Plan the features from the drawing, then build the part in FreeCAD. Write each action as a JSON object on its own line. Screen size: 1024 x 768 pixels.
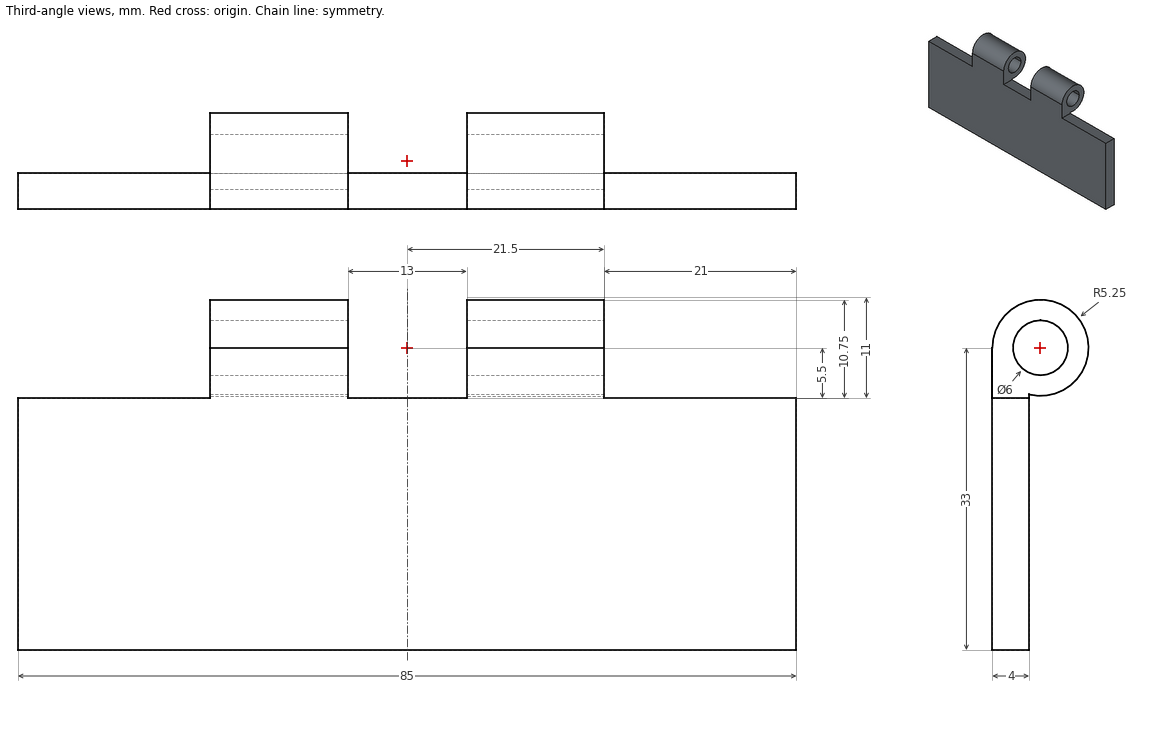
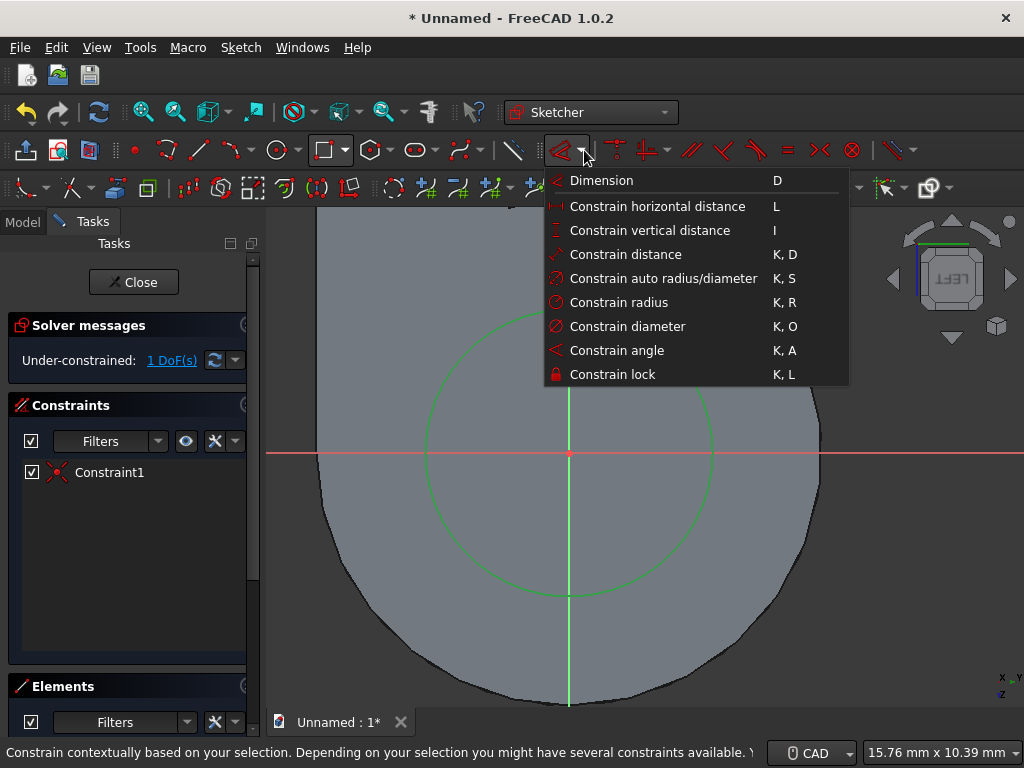
{"action": "left_click", "coordinate": [697, 326]}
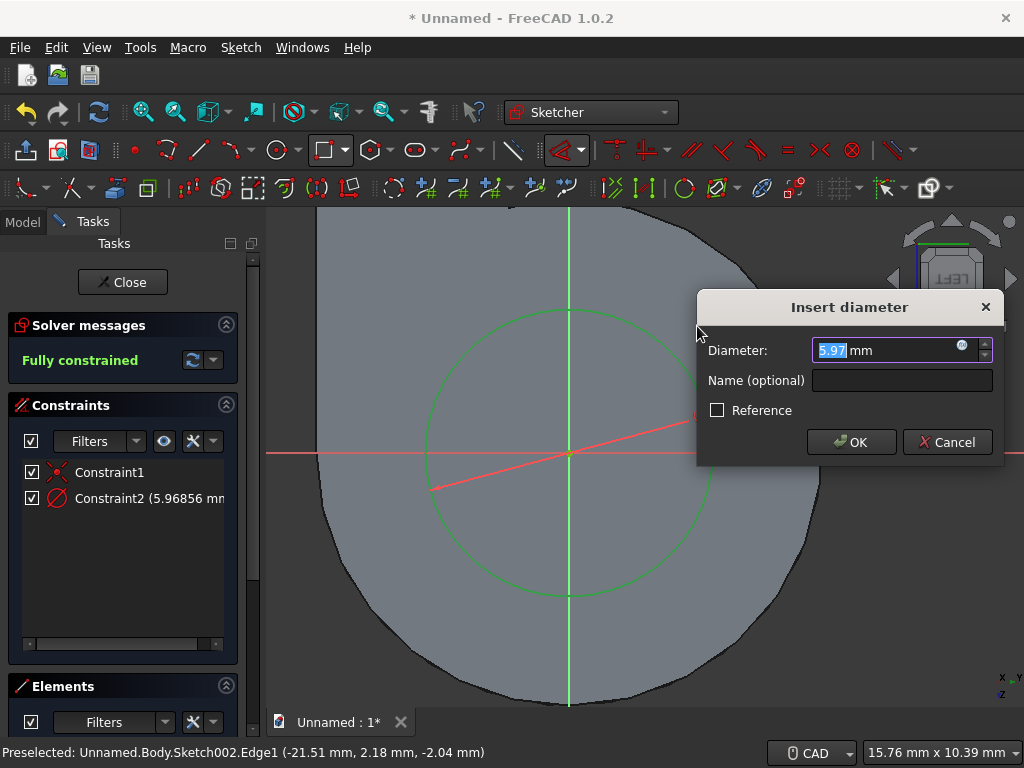
{"action": "type", "text": "6"}
{"action": "key", "text": "Return"}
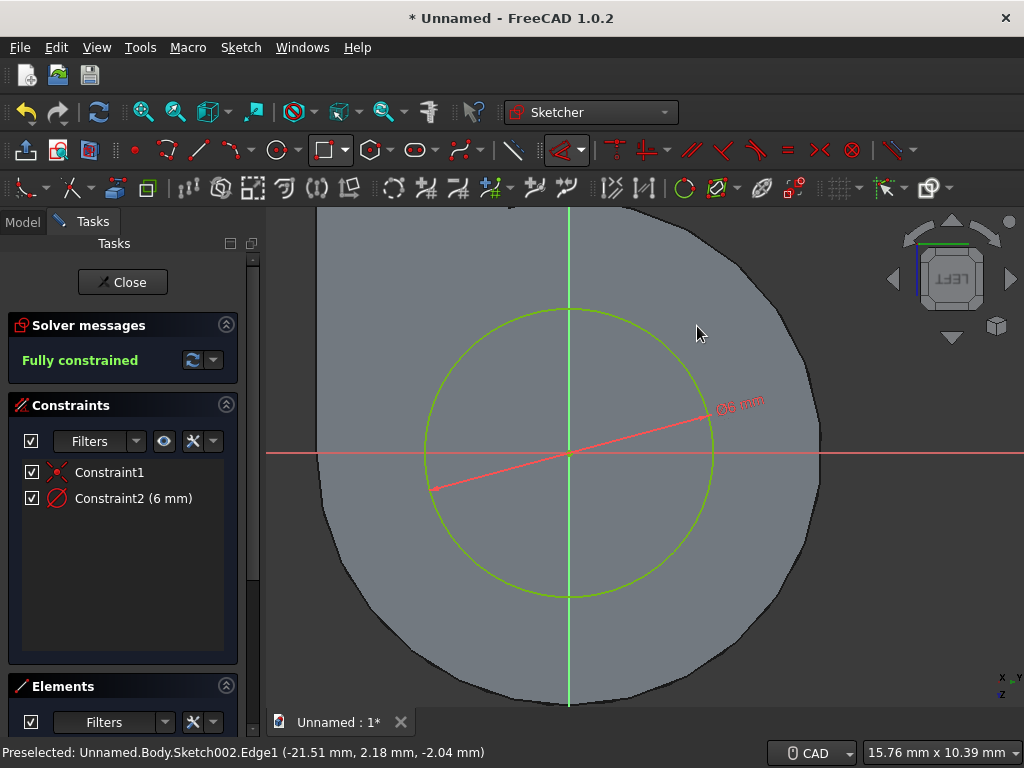
{"action": "left_click", "coordinate": [123, 282]}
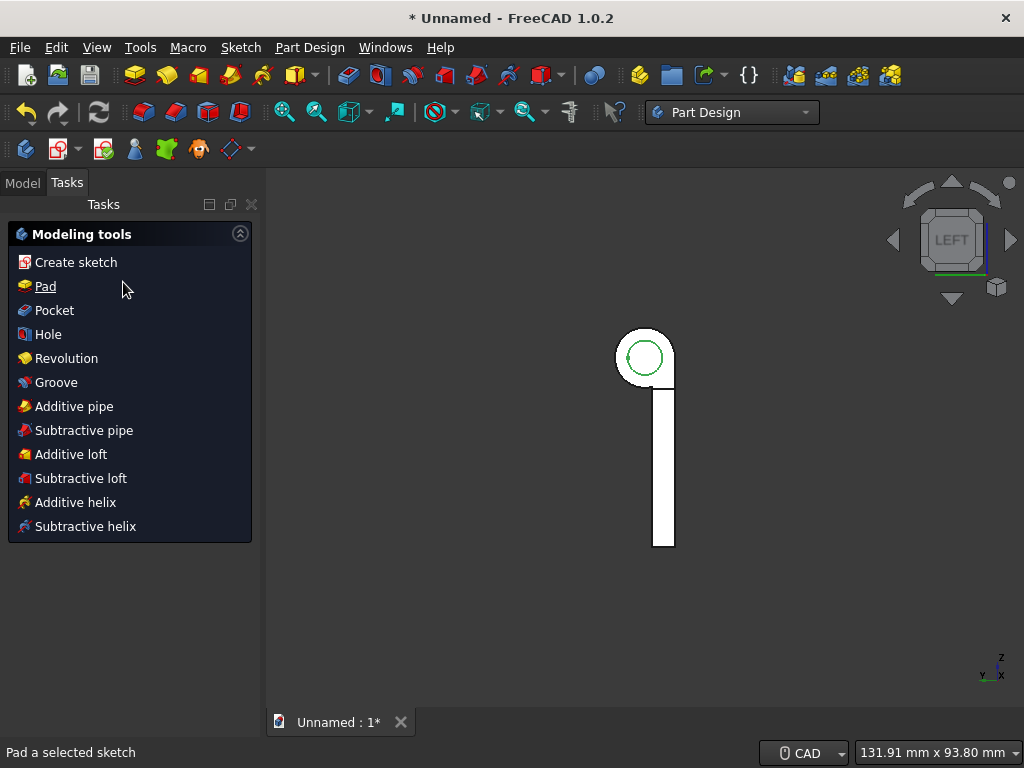
{"action": "left_click", "coordinate": [350, 76]}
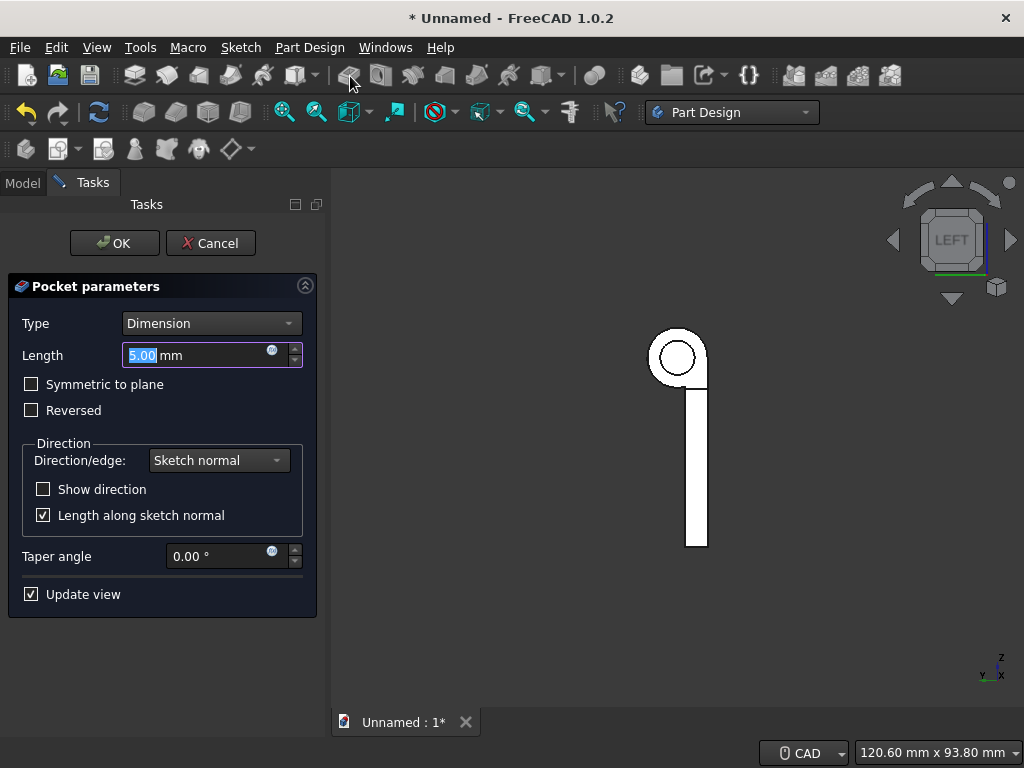
{"action": "left_click", "coordinate": [212, 324]}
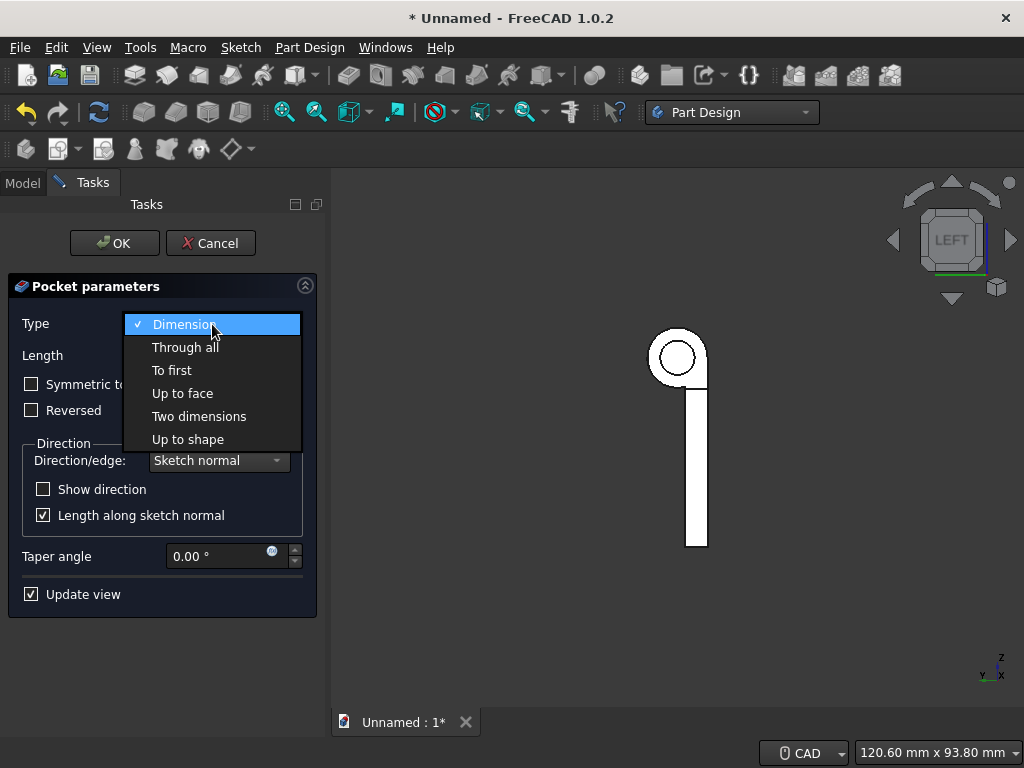
{"action": "left_click", "coordinate": [212, 348]}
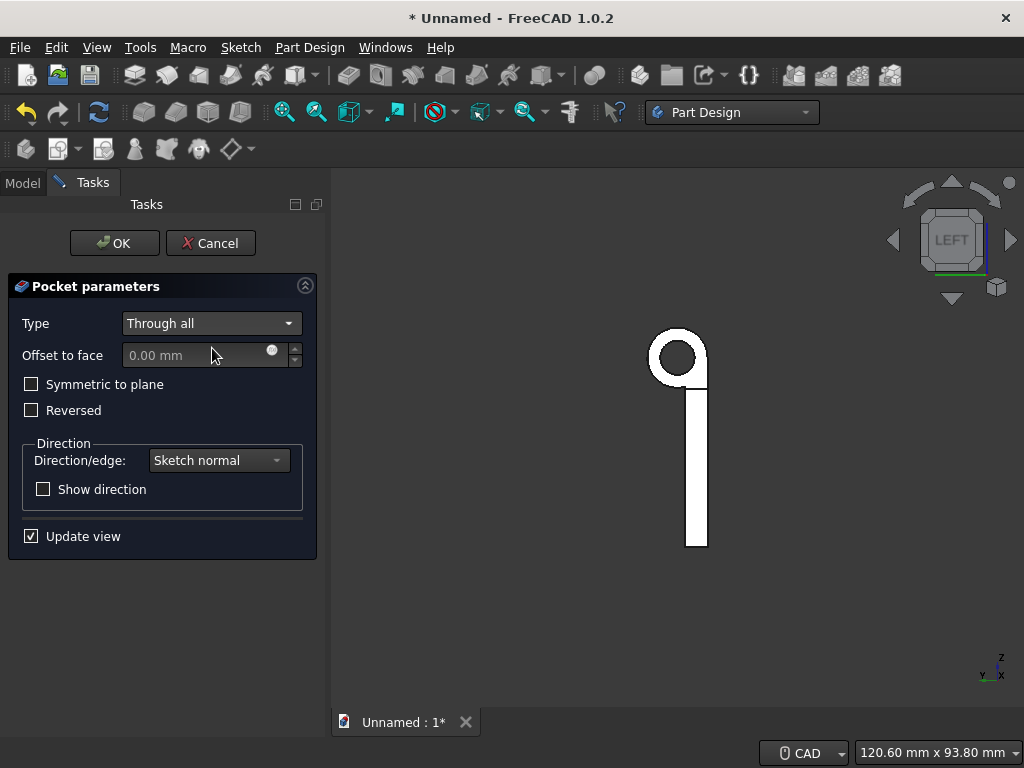
{"action": "left_click", "coordinate": [115, 243]}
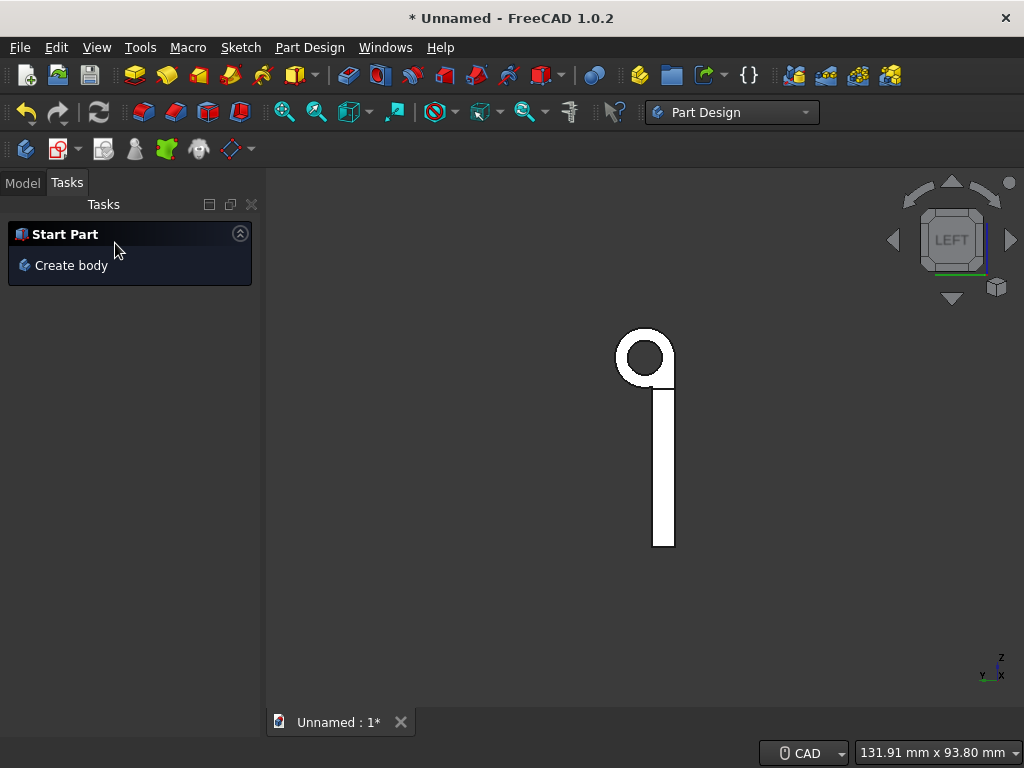
{"action": "key", "text": "0"}